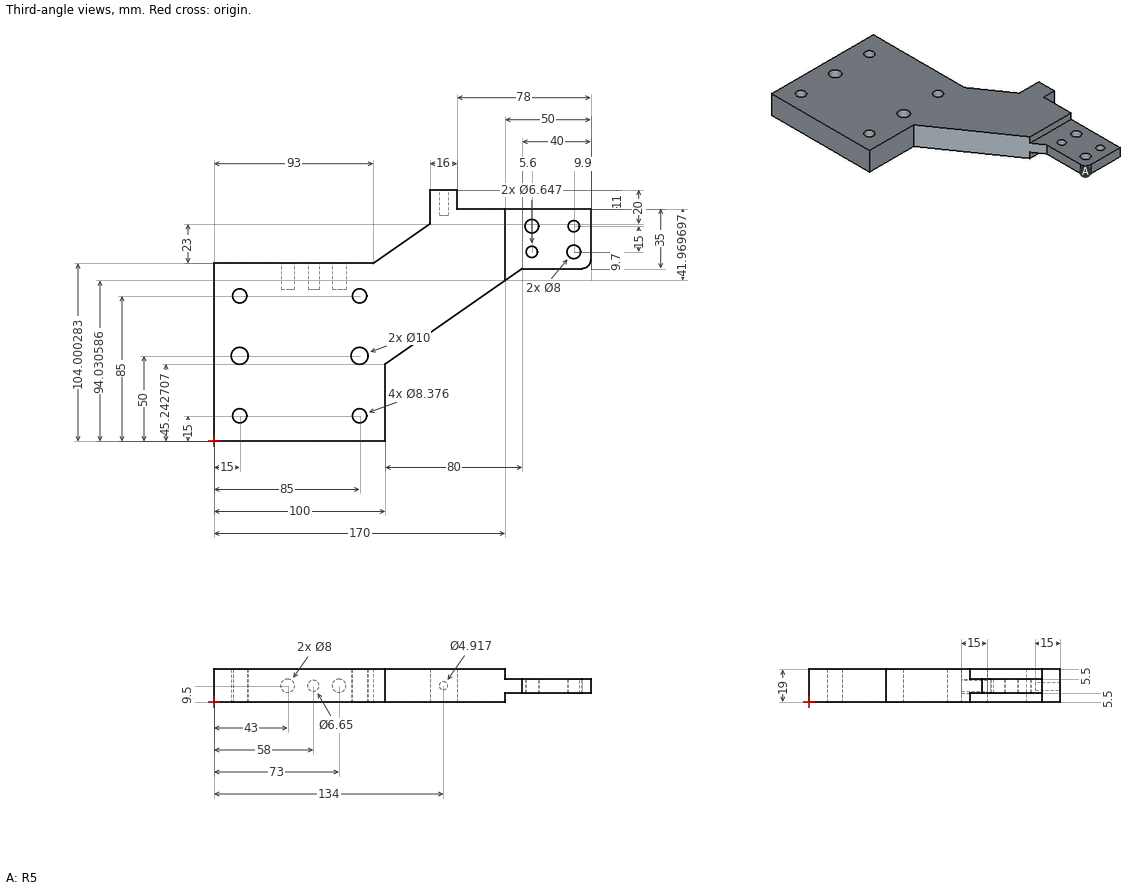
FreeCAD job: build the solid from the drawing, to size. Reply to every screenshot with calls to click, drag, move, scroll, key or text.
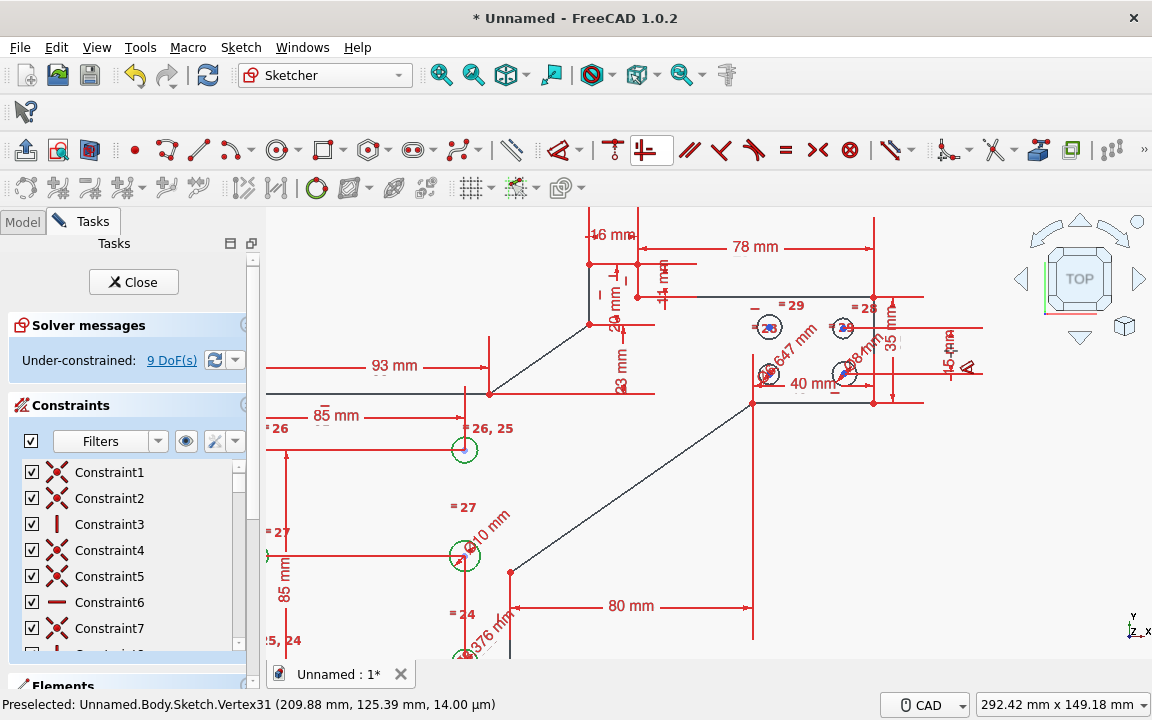
click(769, 374)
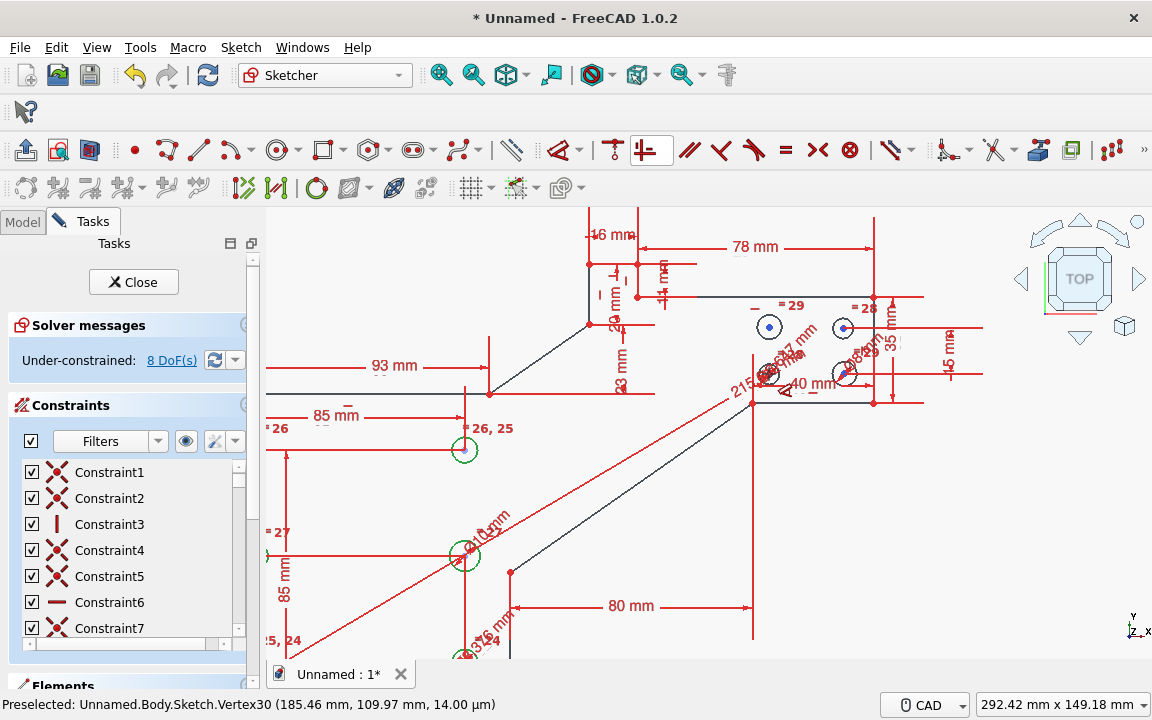
click(843, 328)
click(711, 351)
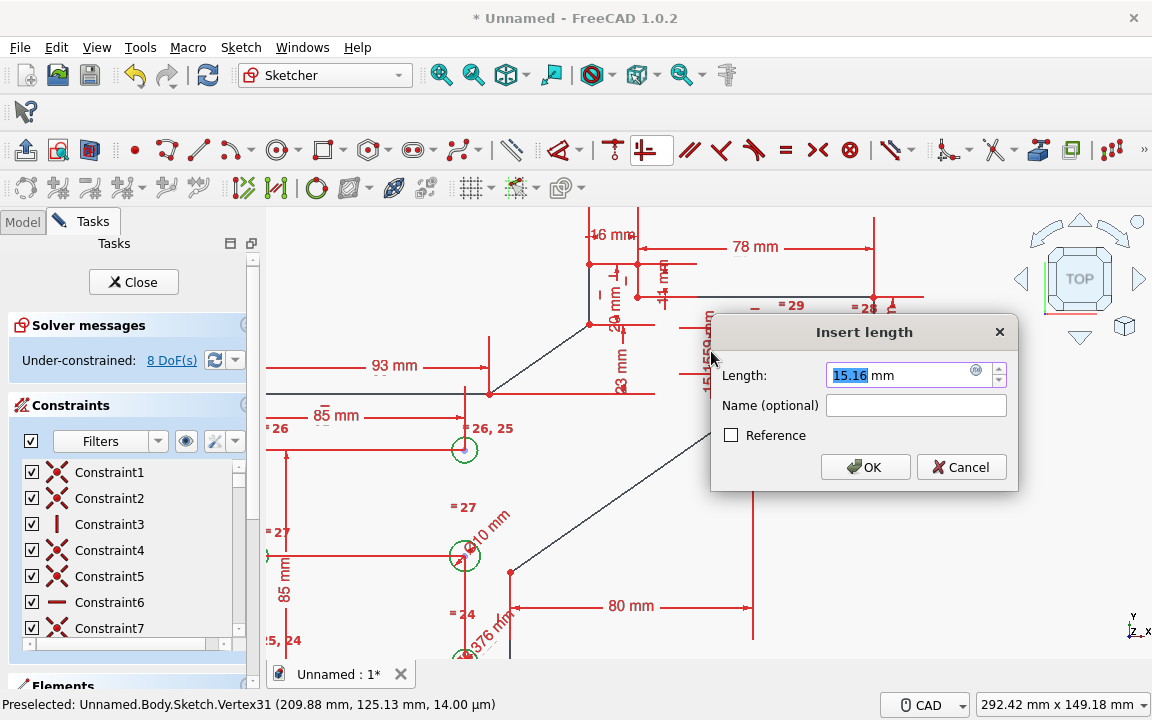
text(15)
key(Return)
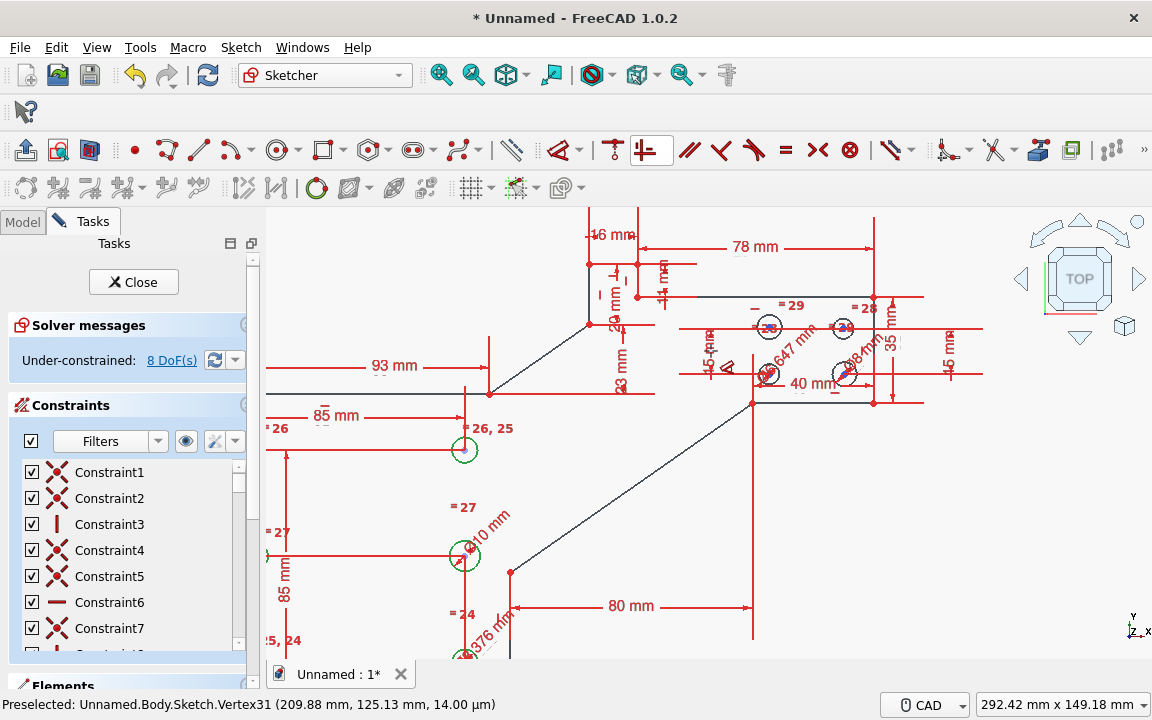
click(769, 374)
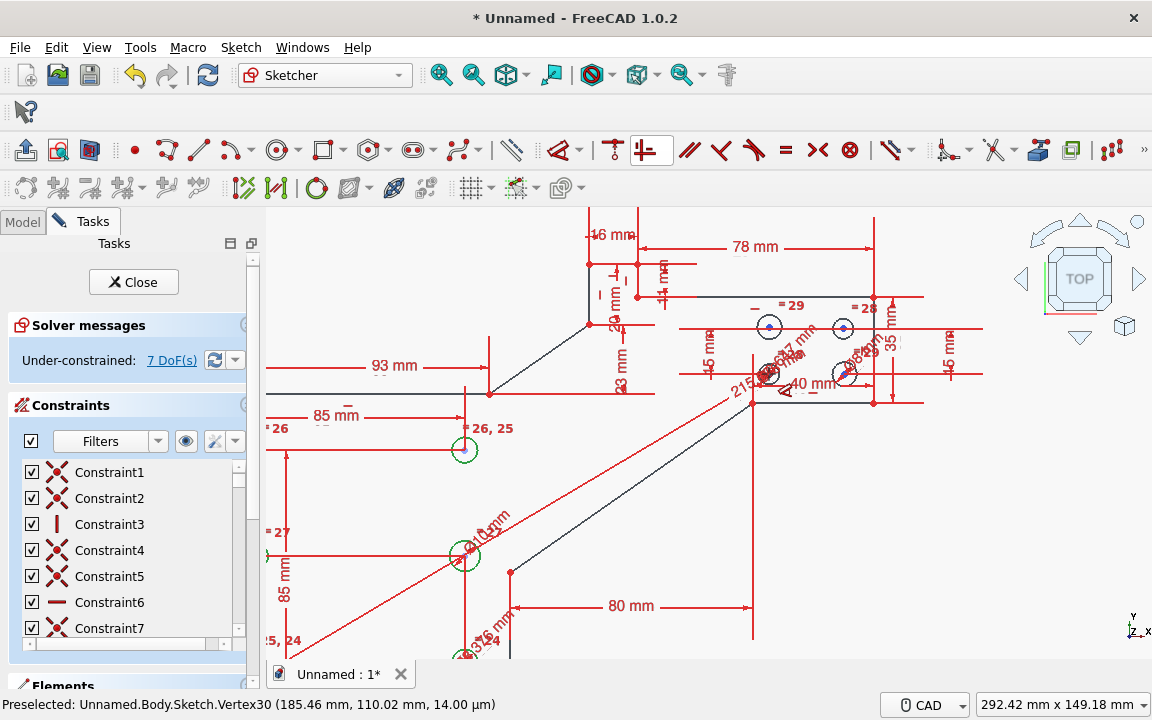
click(770, 327)
click(639, 340)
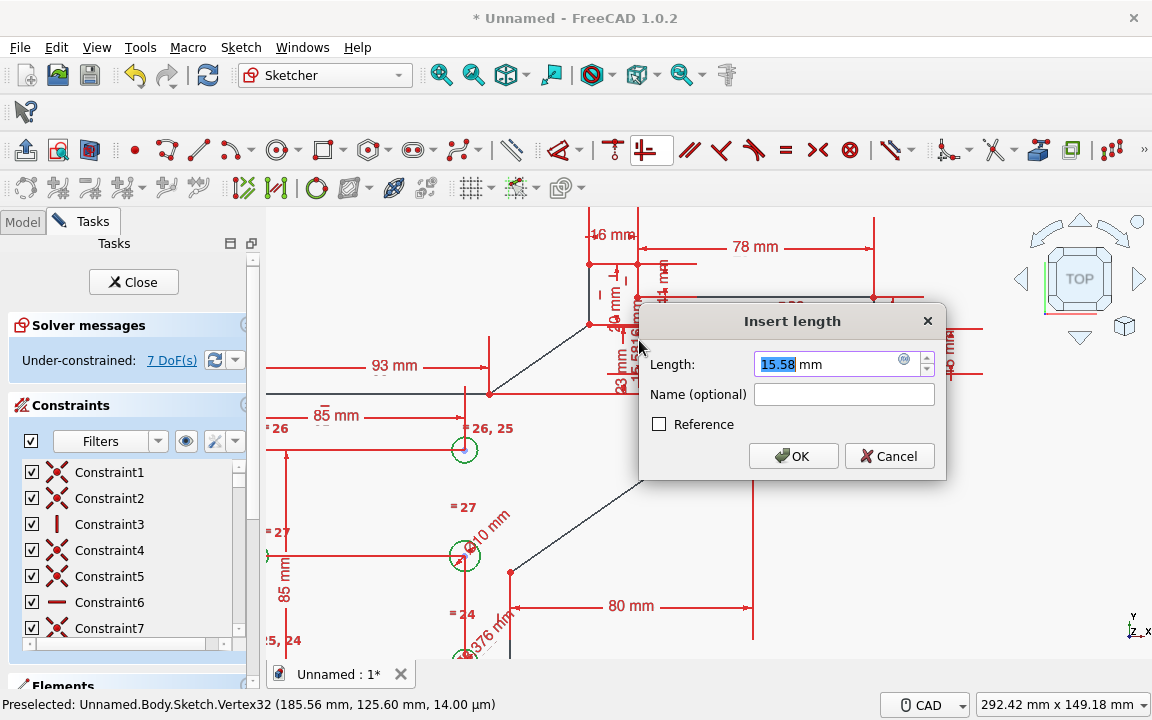
text(15)
key(Return)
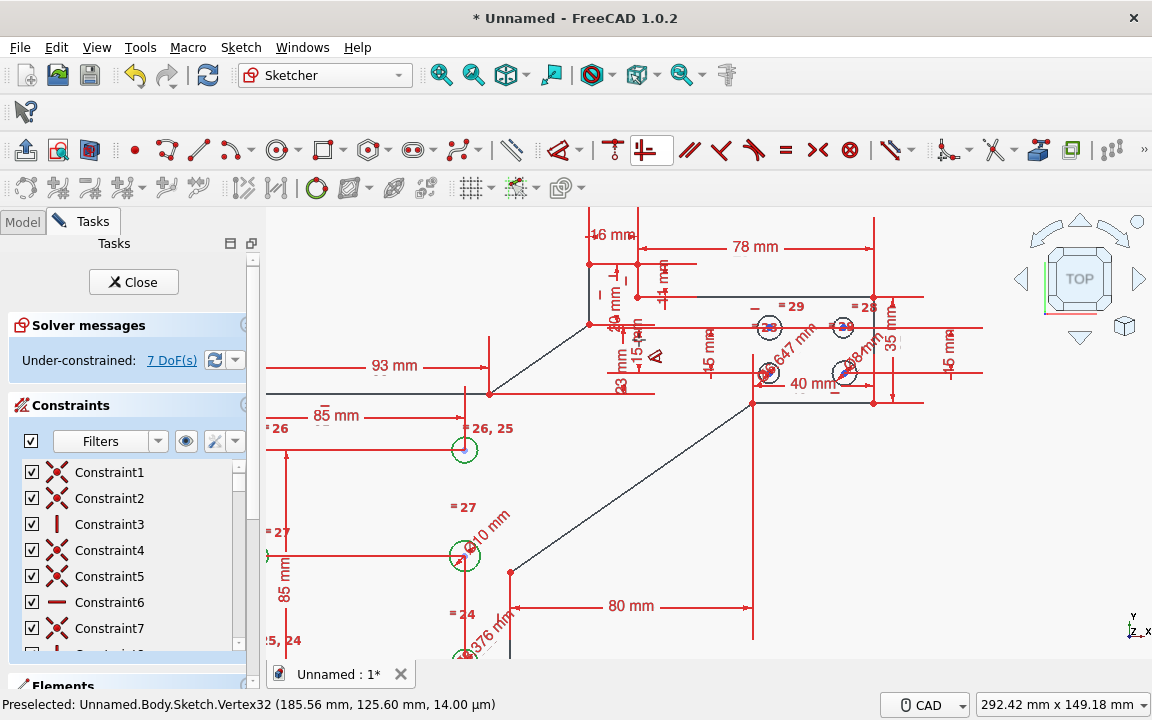
scroll(874, 403, up, 2)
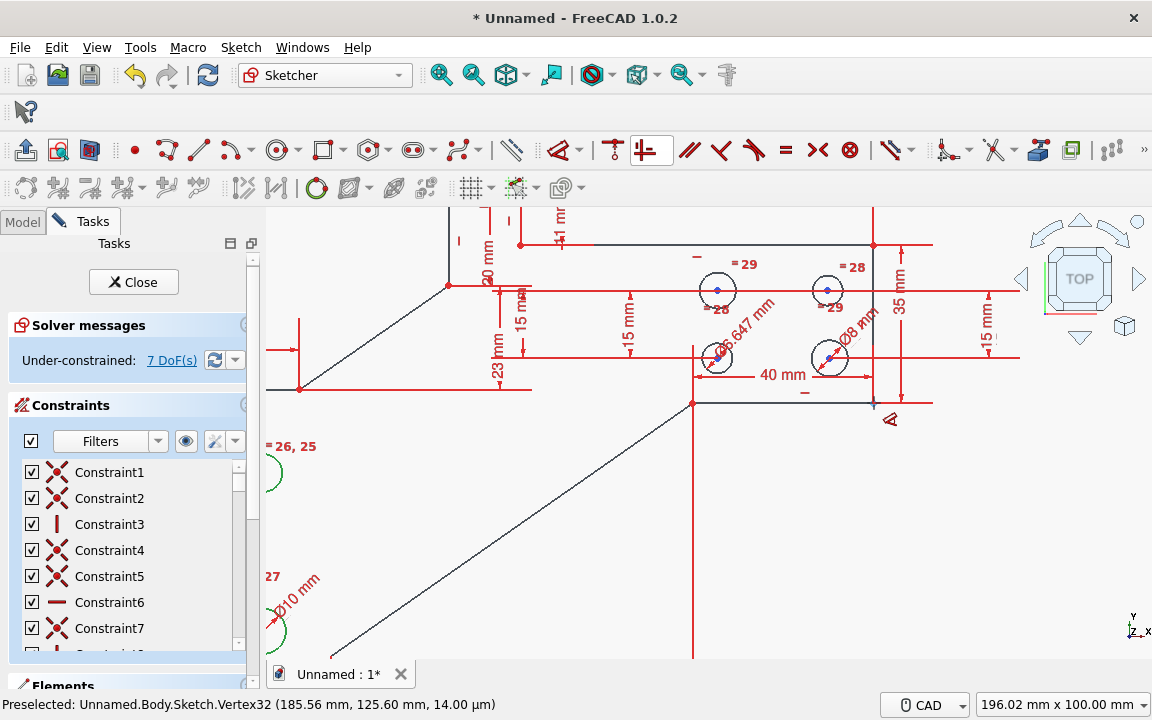
click(873, 403)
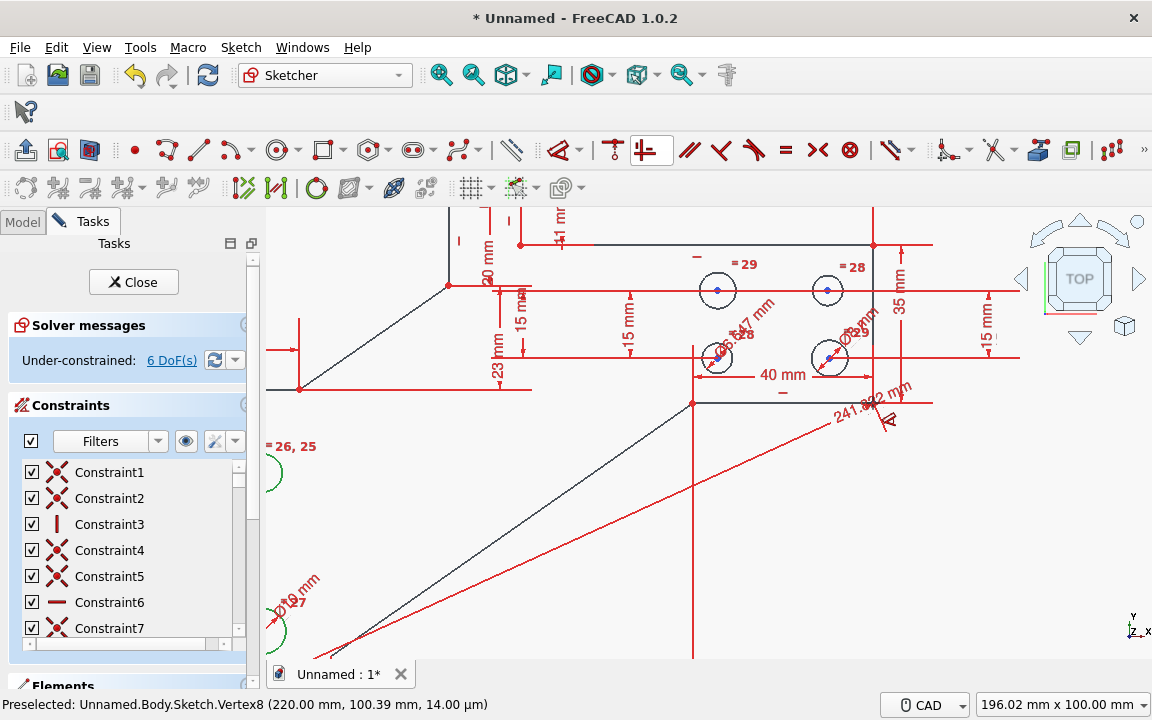
click(830, 358)
click(852, 437)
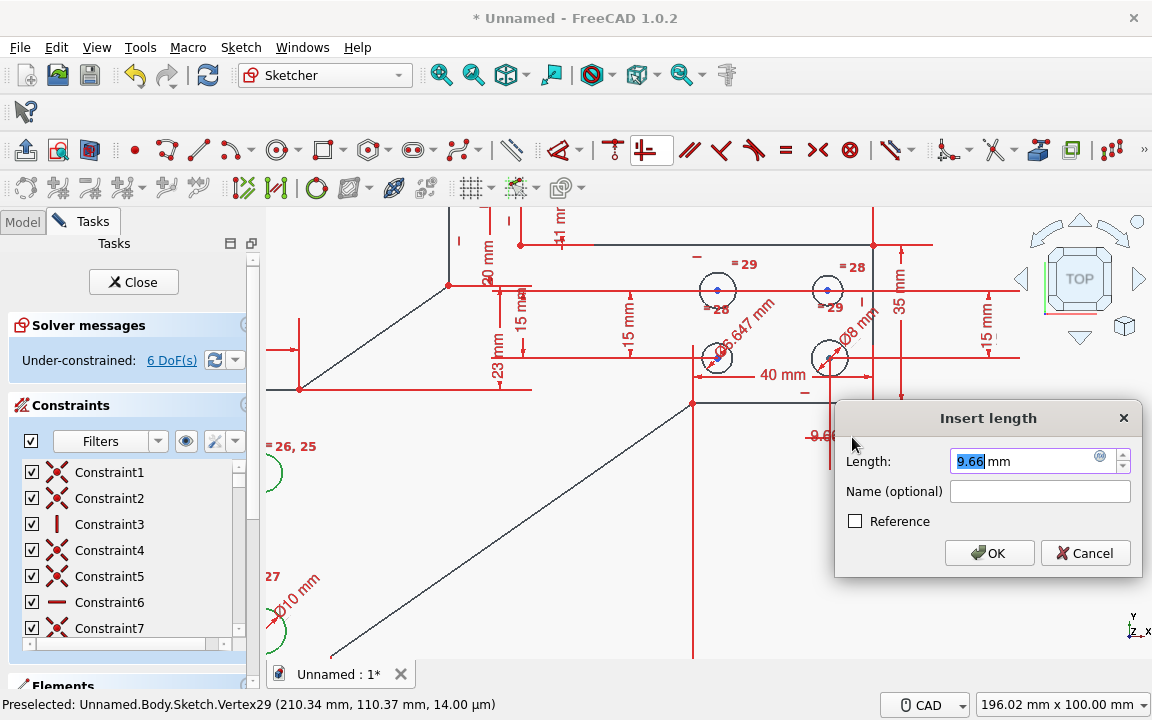
text(9.9)
key(Return)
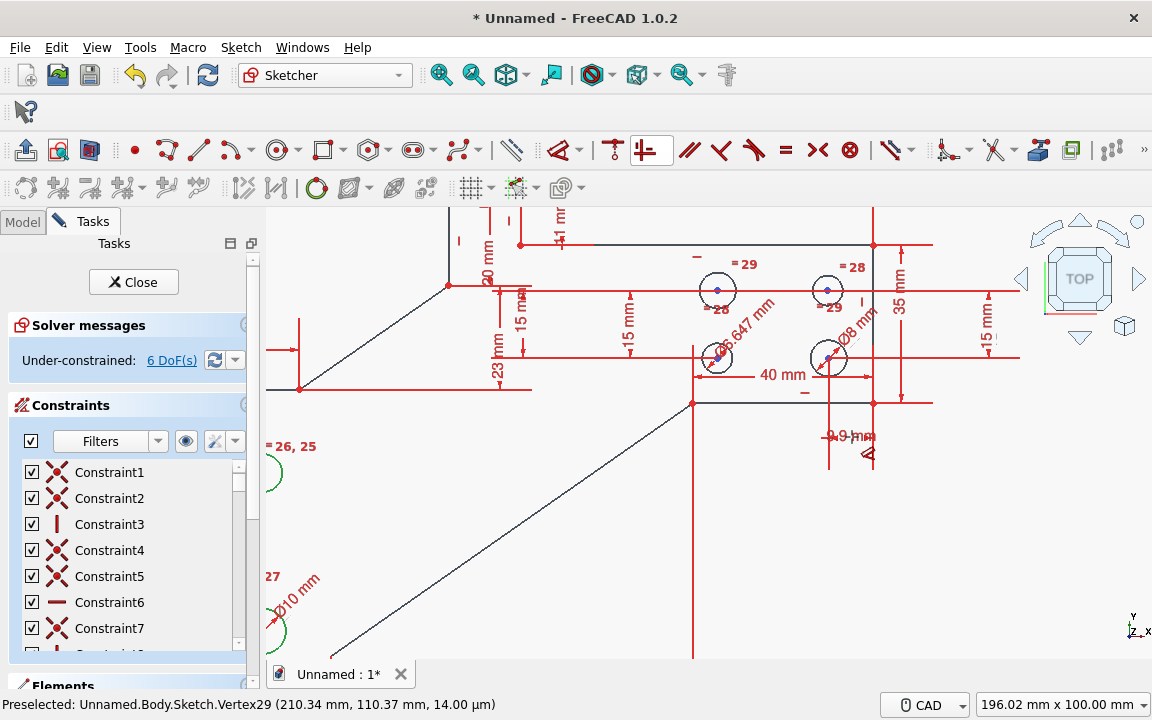
click(873, 403)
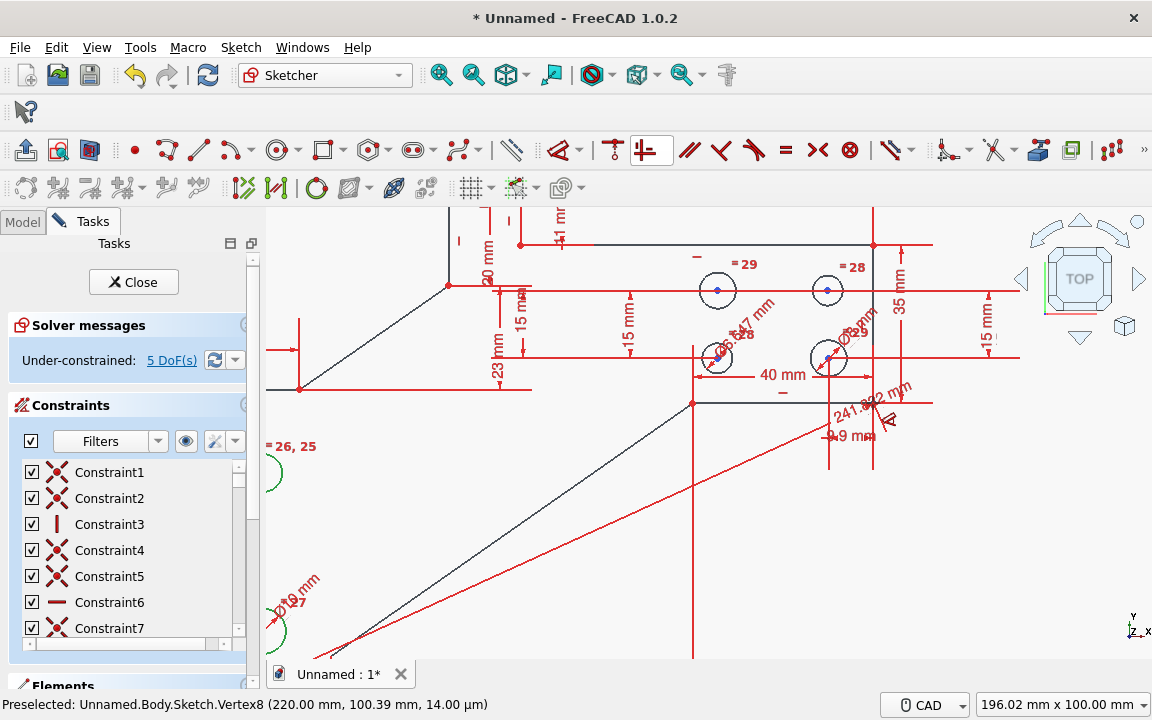
click(829, 358)
click(907, 381)